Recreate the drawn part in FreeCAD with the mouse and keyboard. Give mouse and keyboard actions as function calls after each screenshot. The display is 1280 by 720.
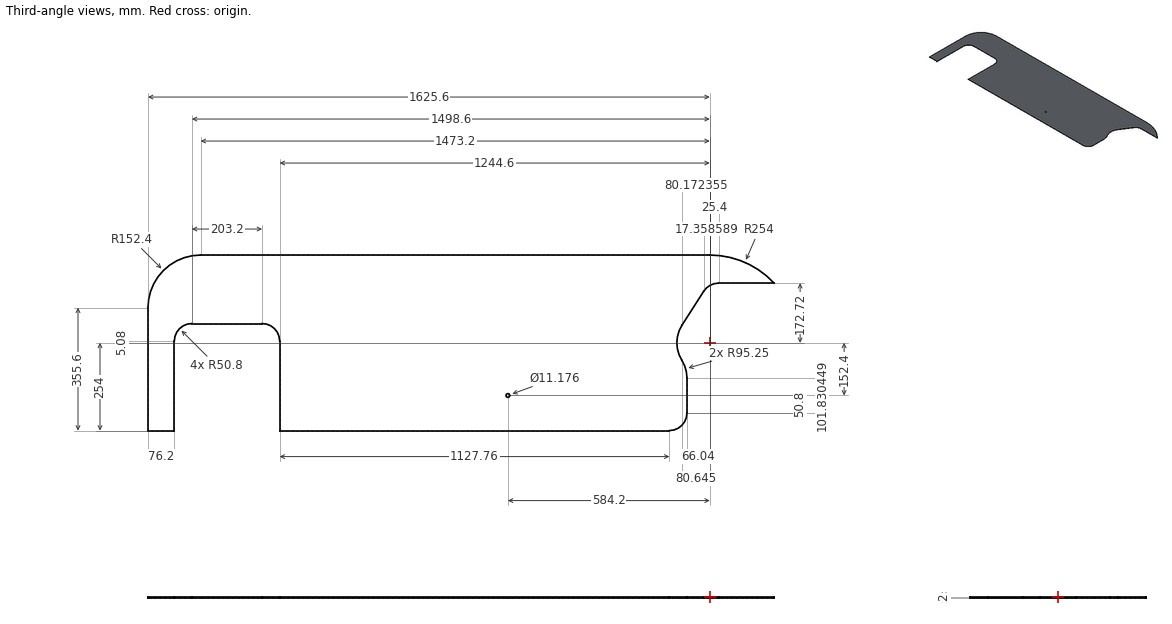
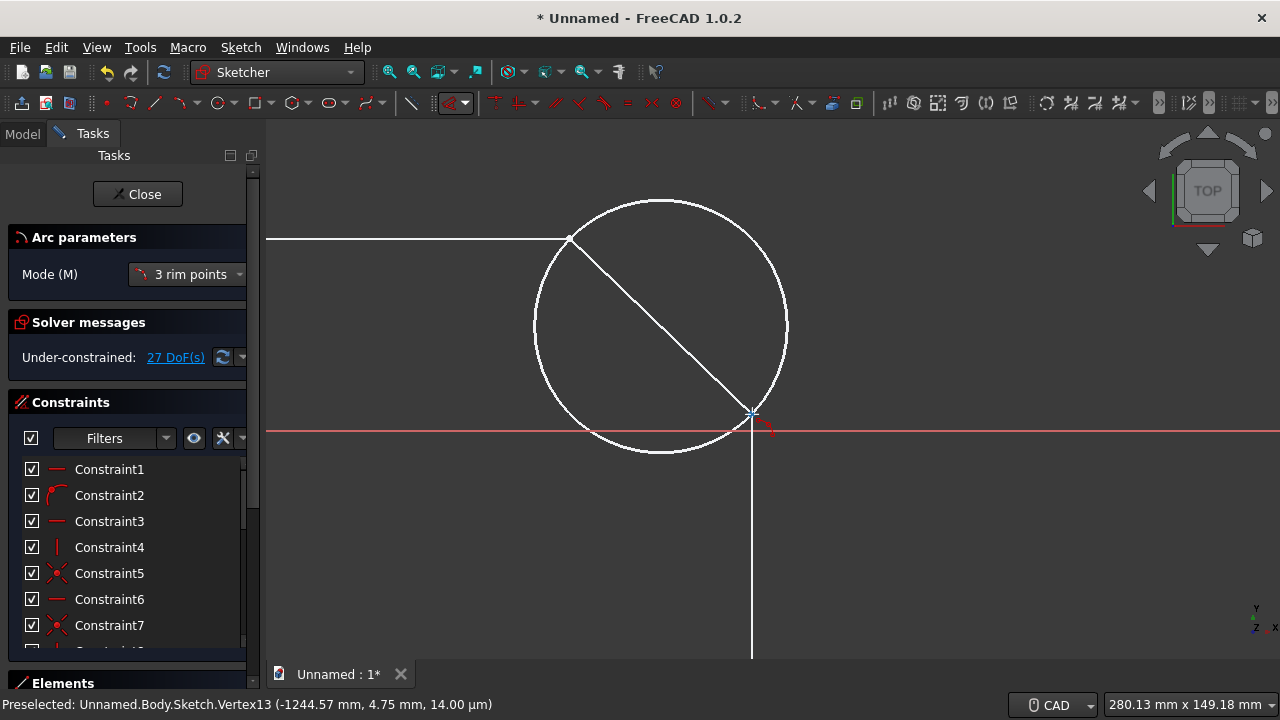
scroll(510, 385, down, 12)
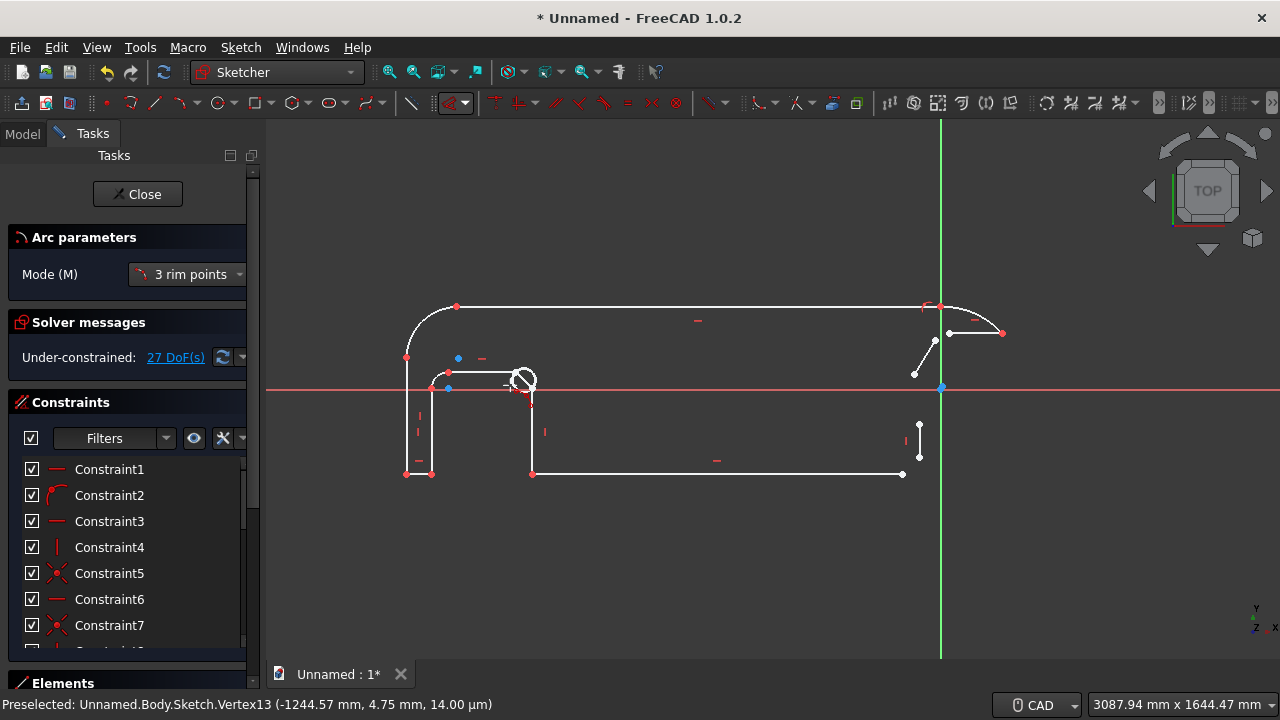
scroll(527, 376, up, 6)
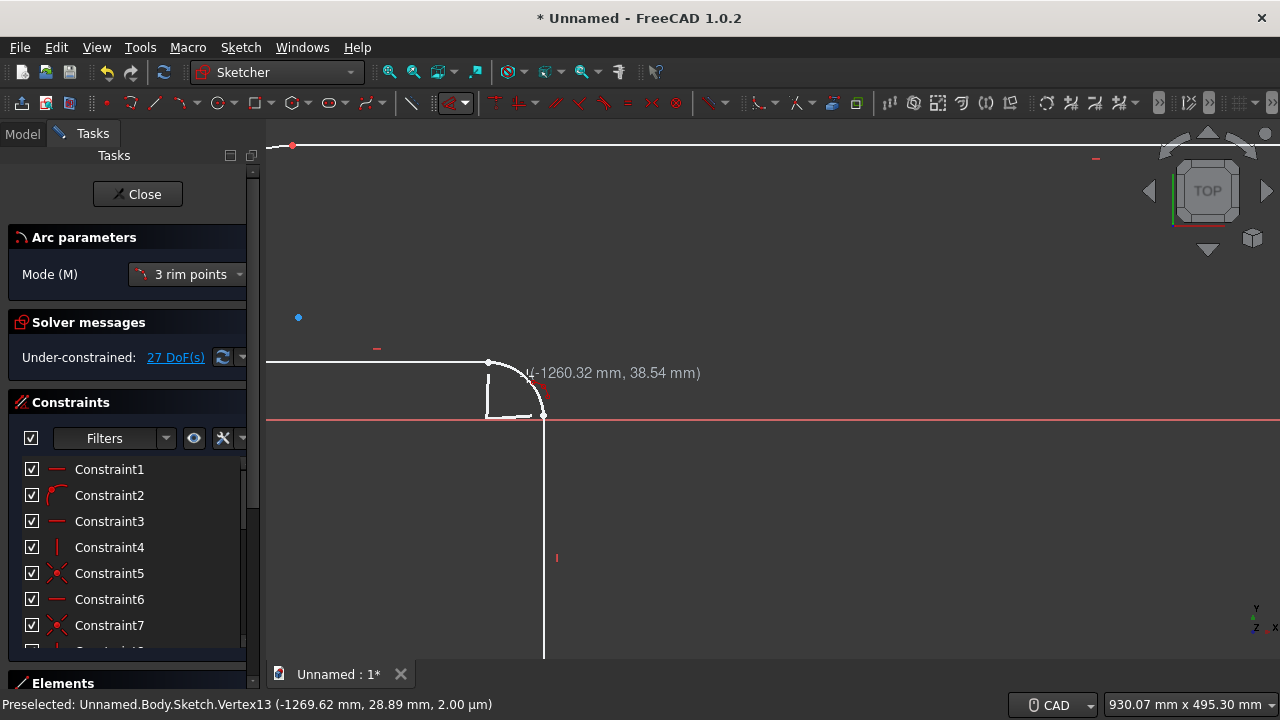
click(527, 376)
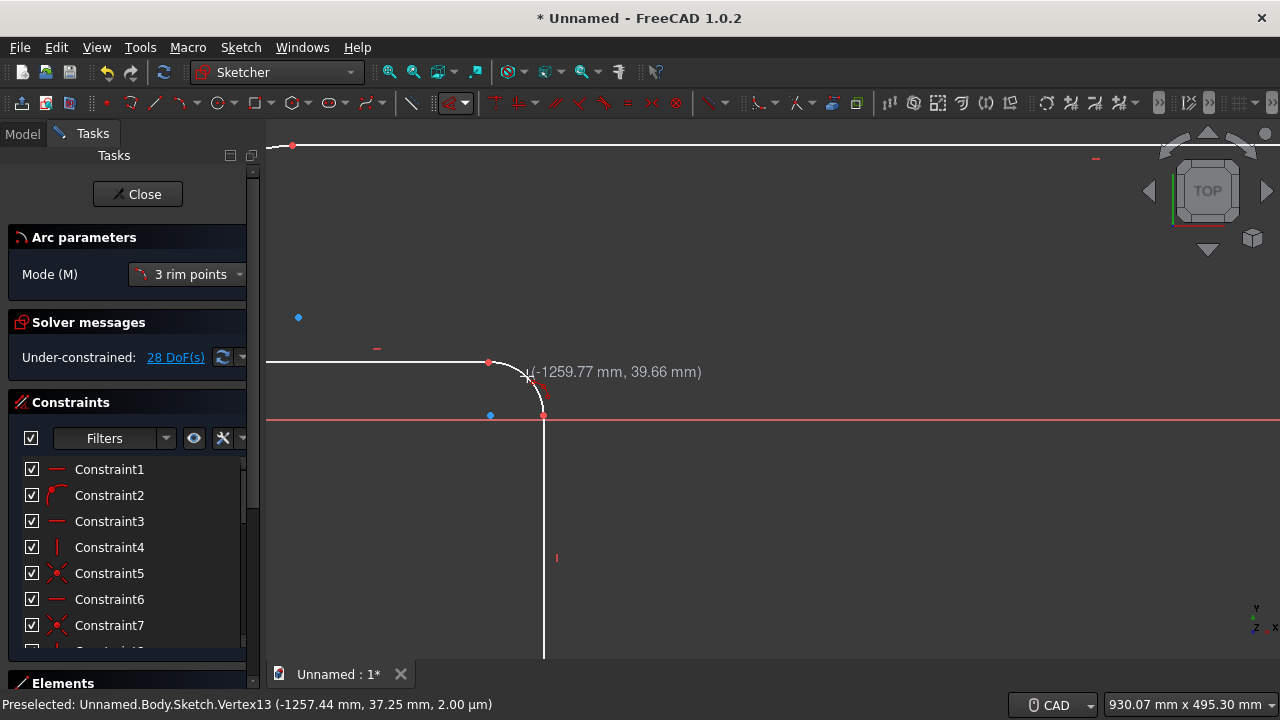
scroll(527, 376, down, 6)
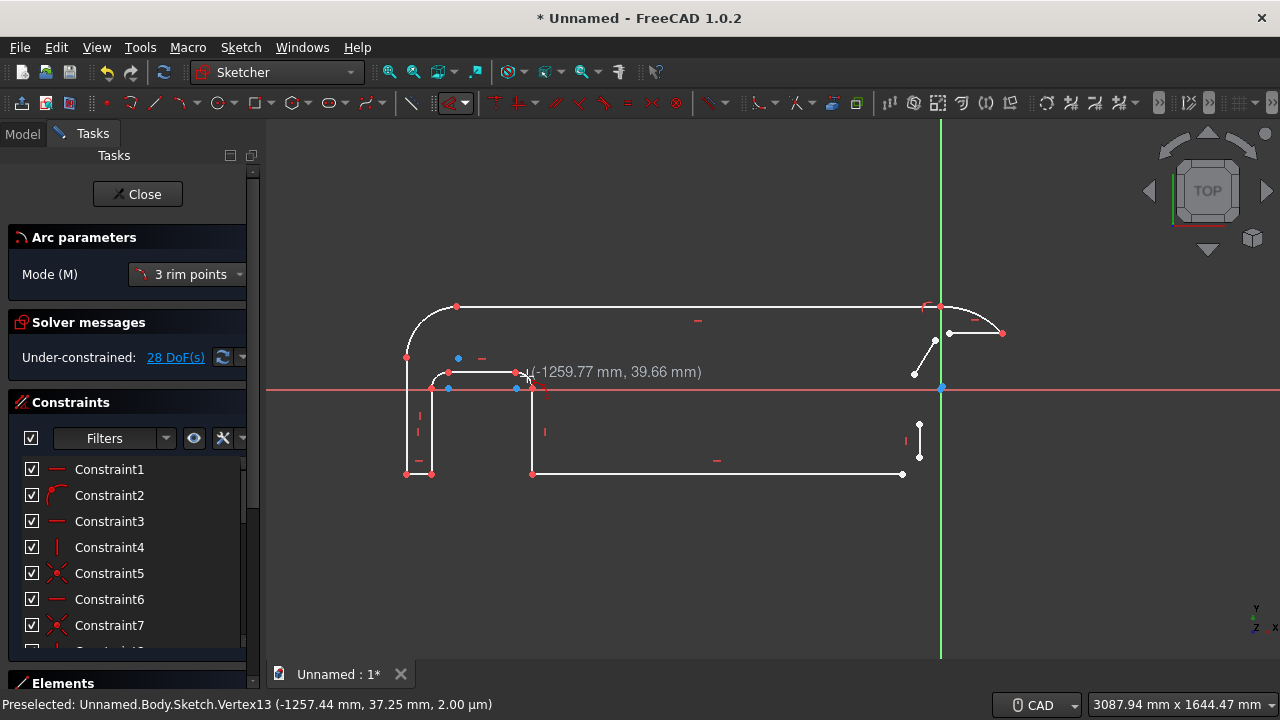
click(903, 474)
click(920, 457)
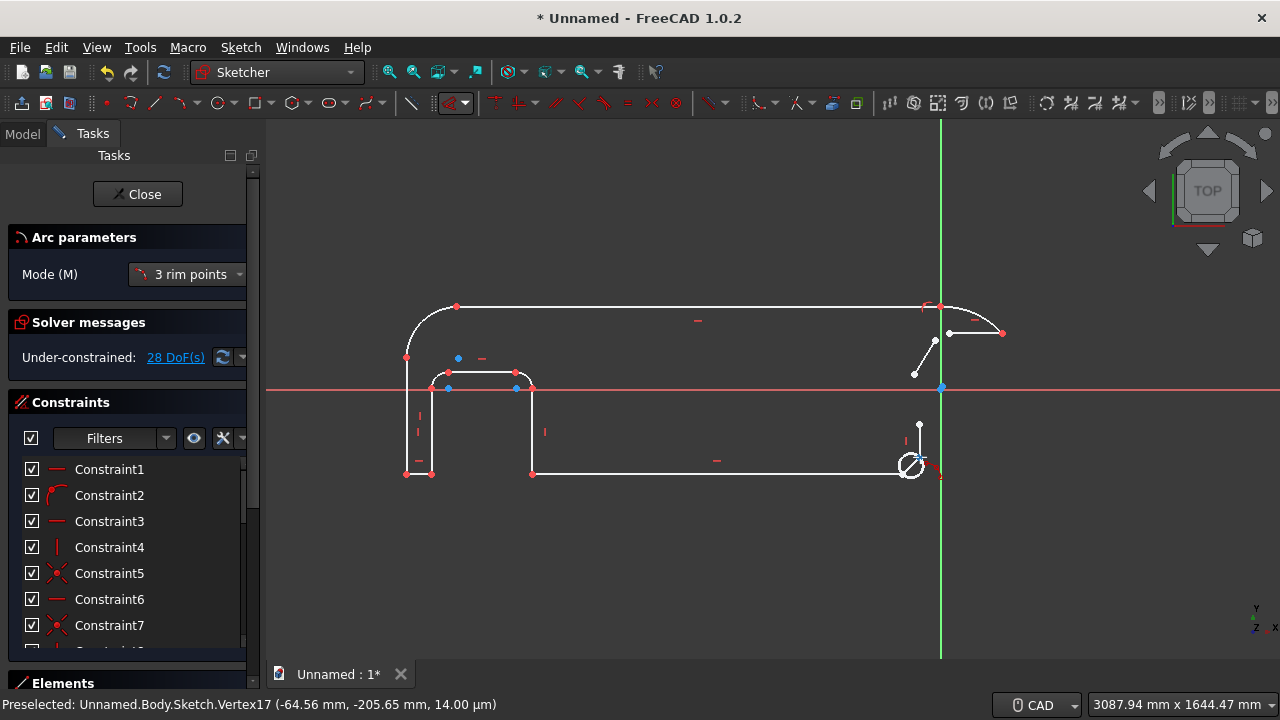
scroll(914, 468, up, 6)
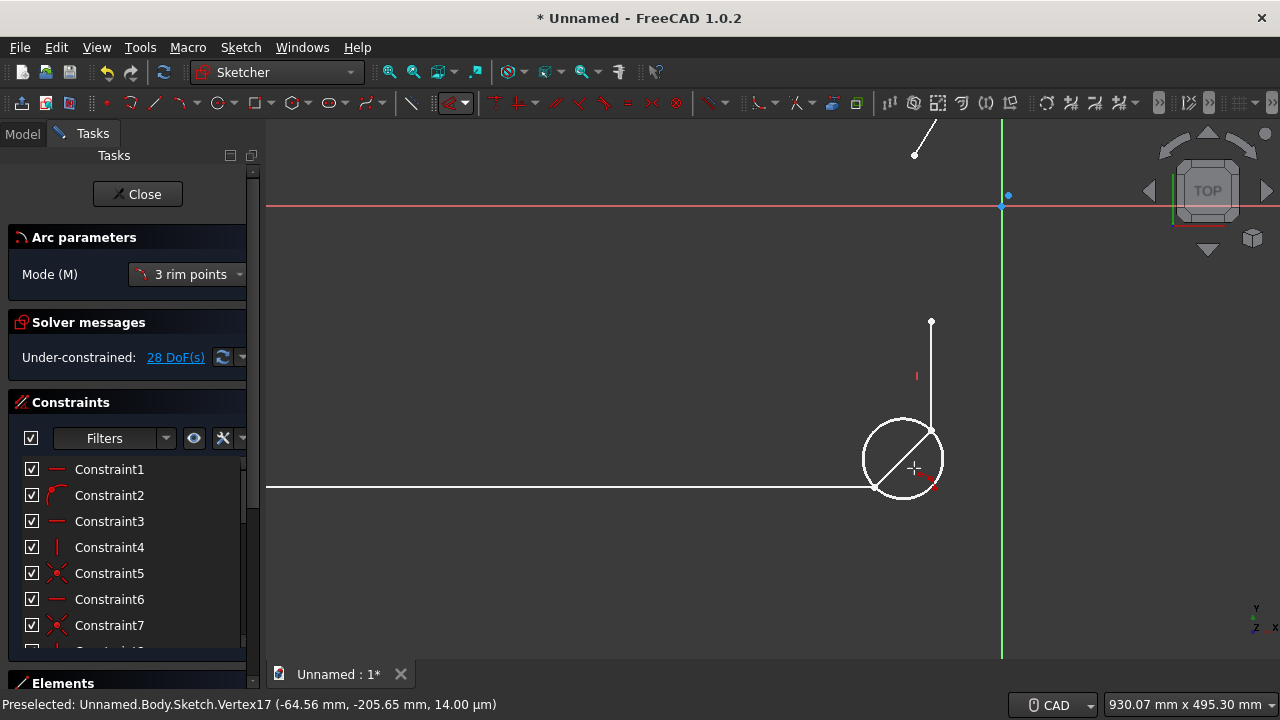
click(913, 467)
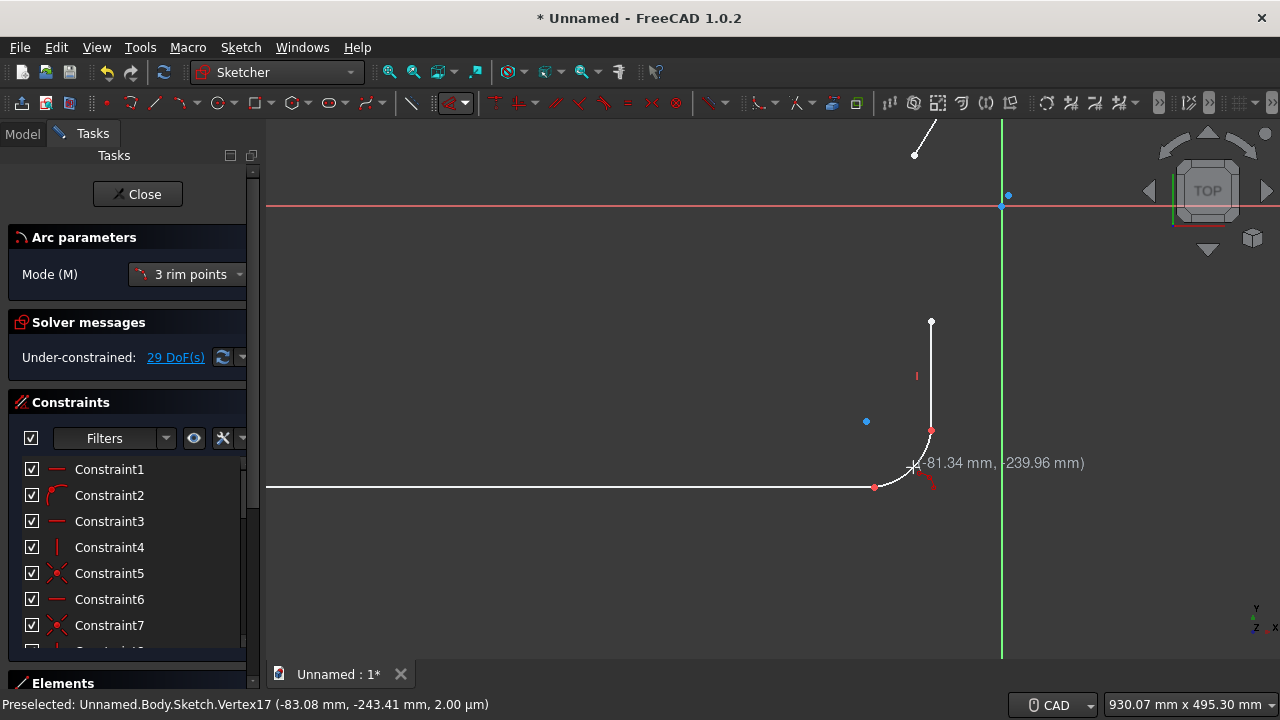
click(931, 321)
click(914, 262)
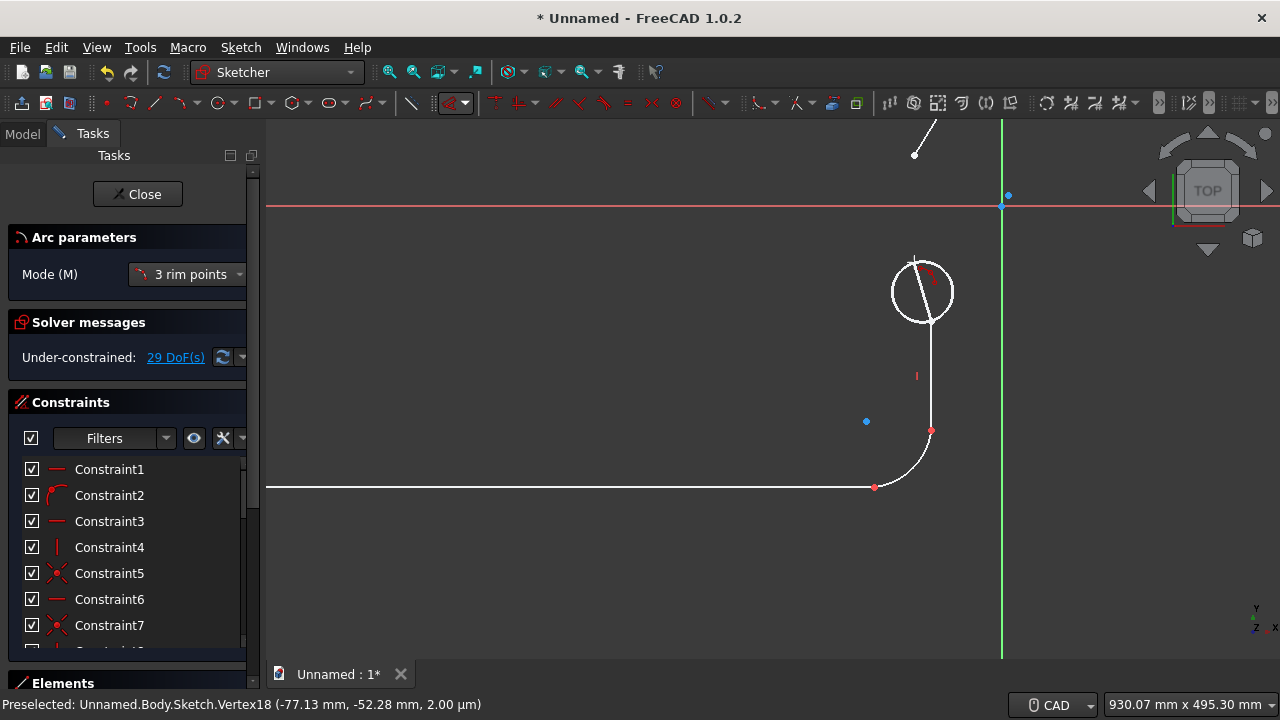
scroll(926, 288, up, 7)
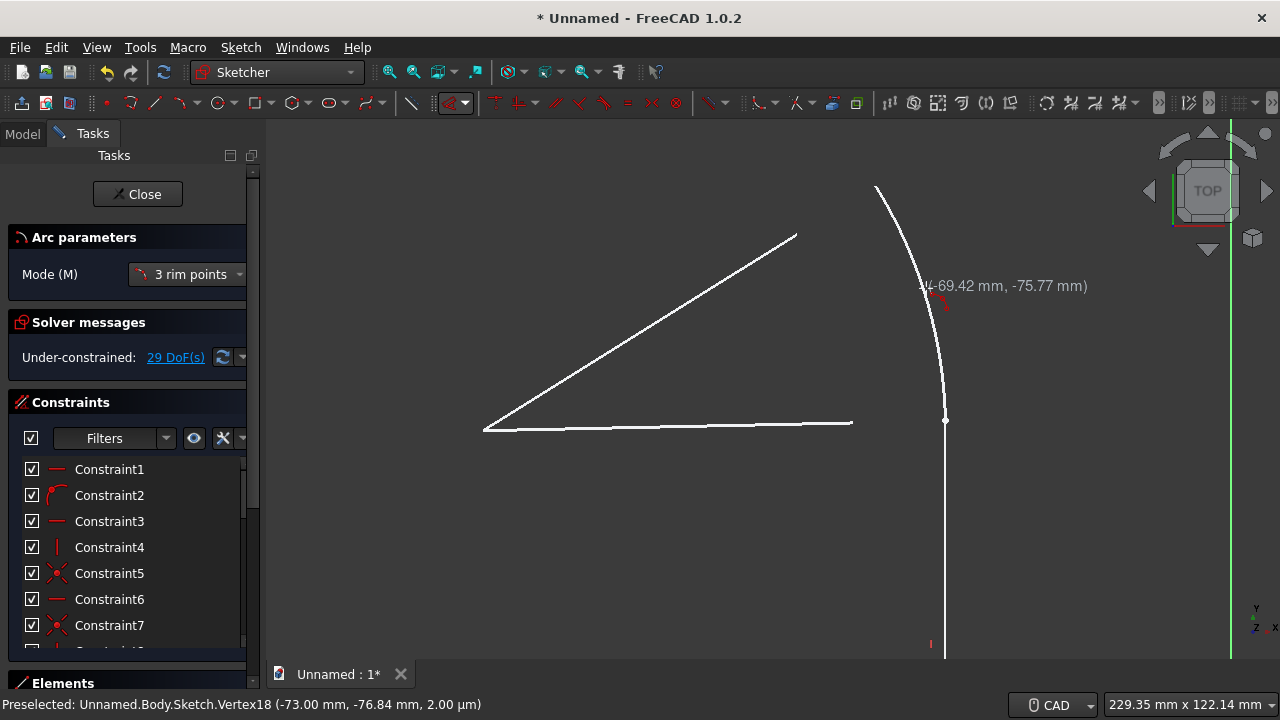
click(922, 288)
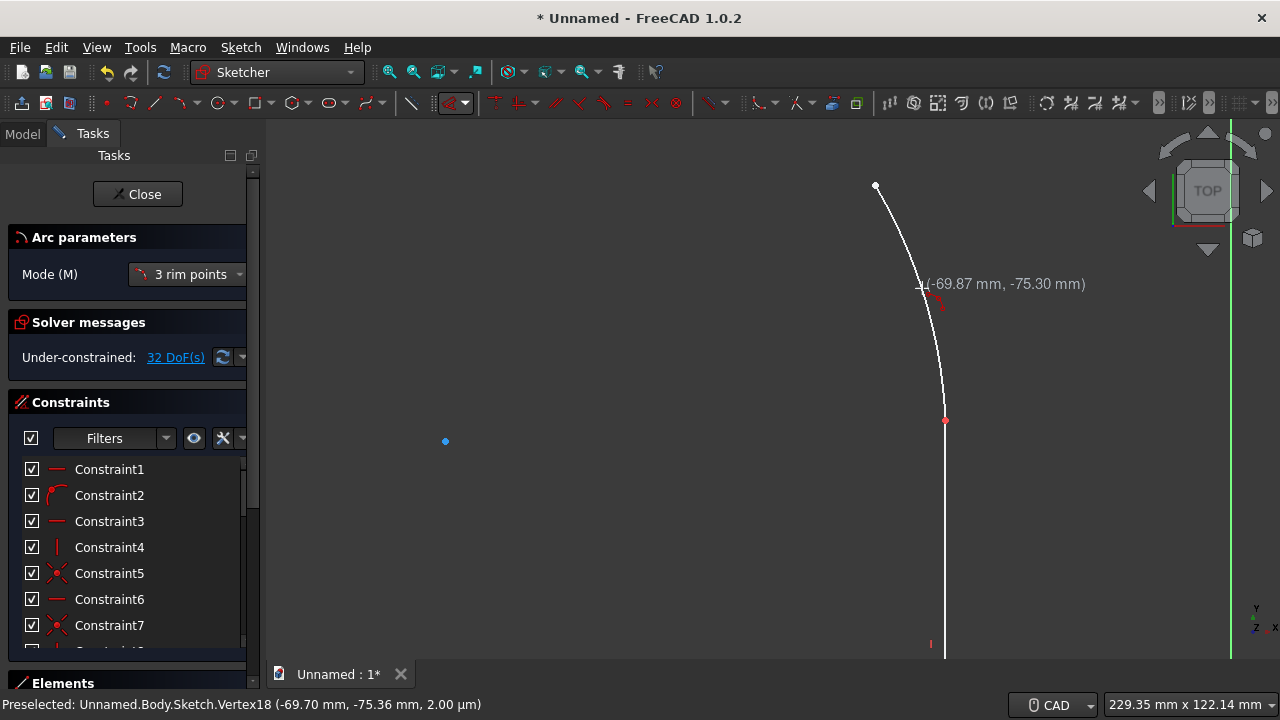
scroll(918, 424, down, 13)